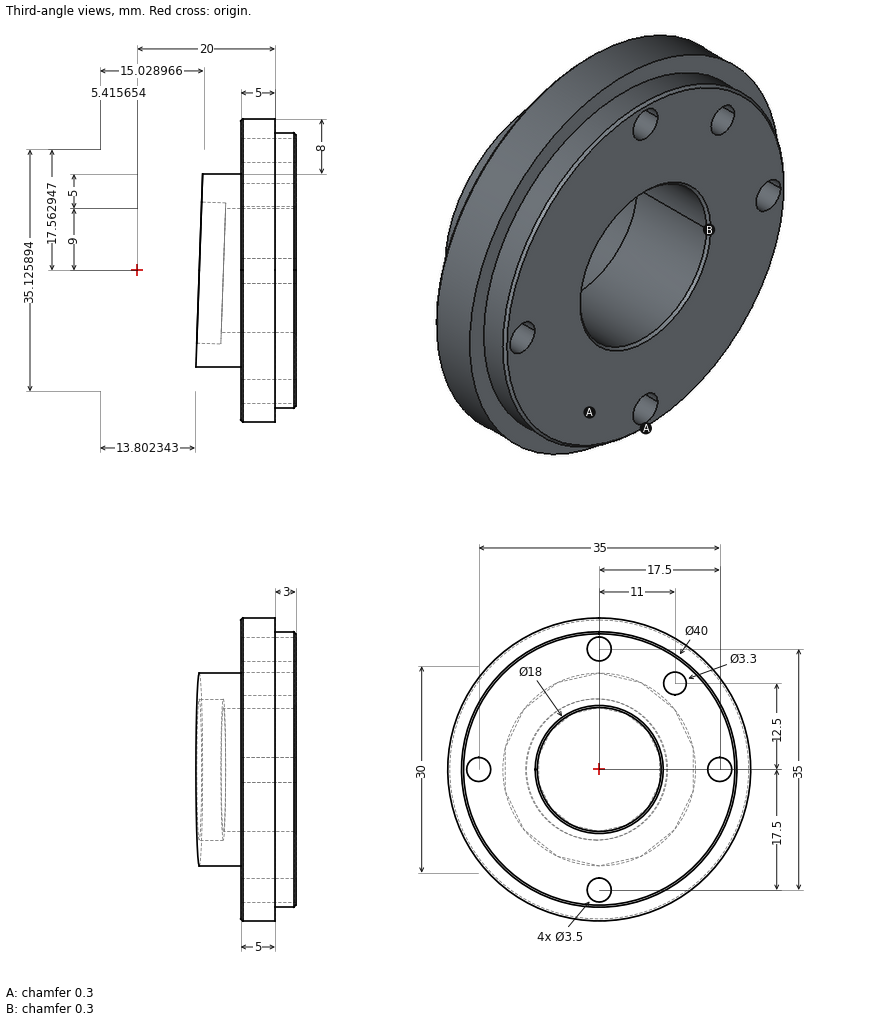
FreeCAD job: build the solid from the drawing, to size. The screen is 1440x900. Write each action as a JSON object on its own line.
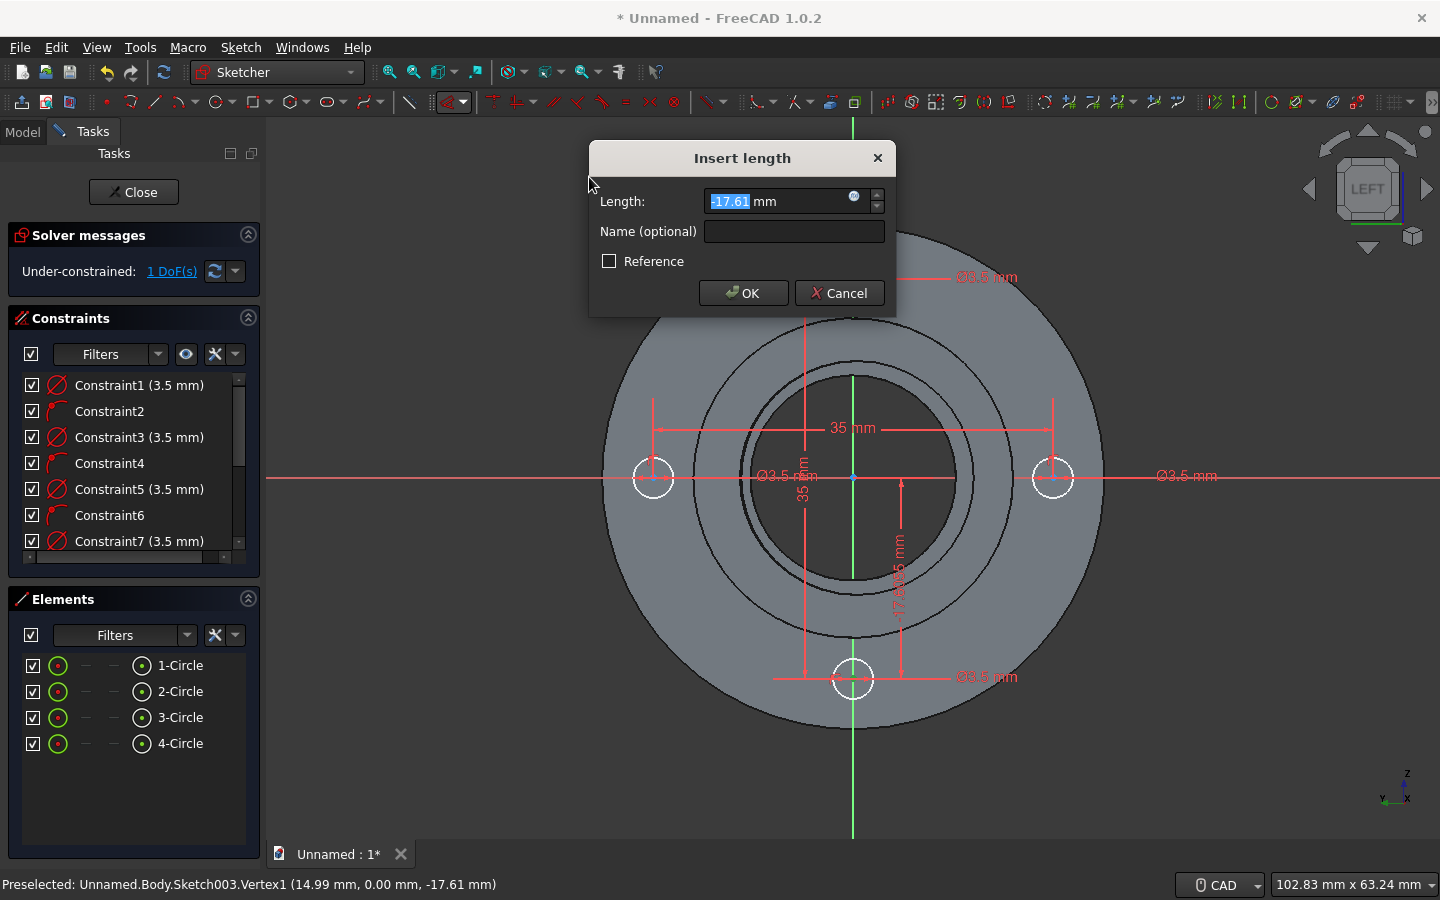
{"action": "type", "text": "-17.5"}
{"action": "key", "text": "Return"}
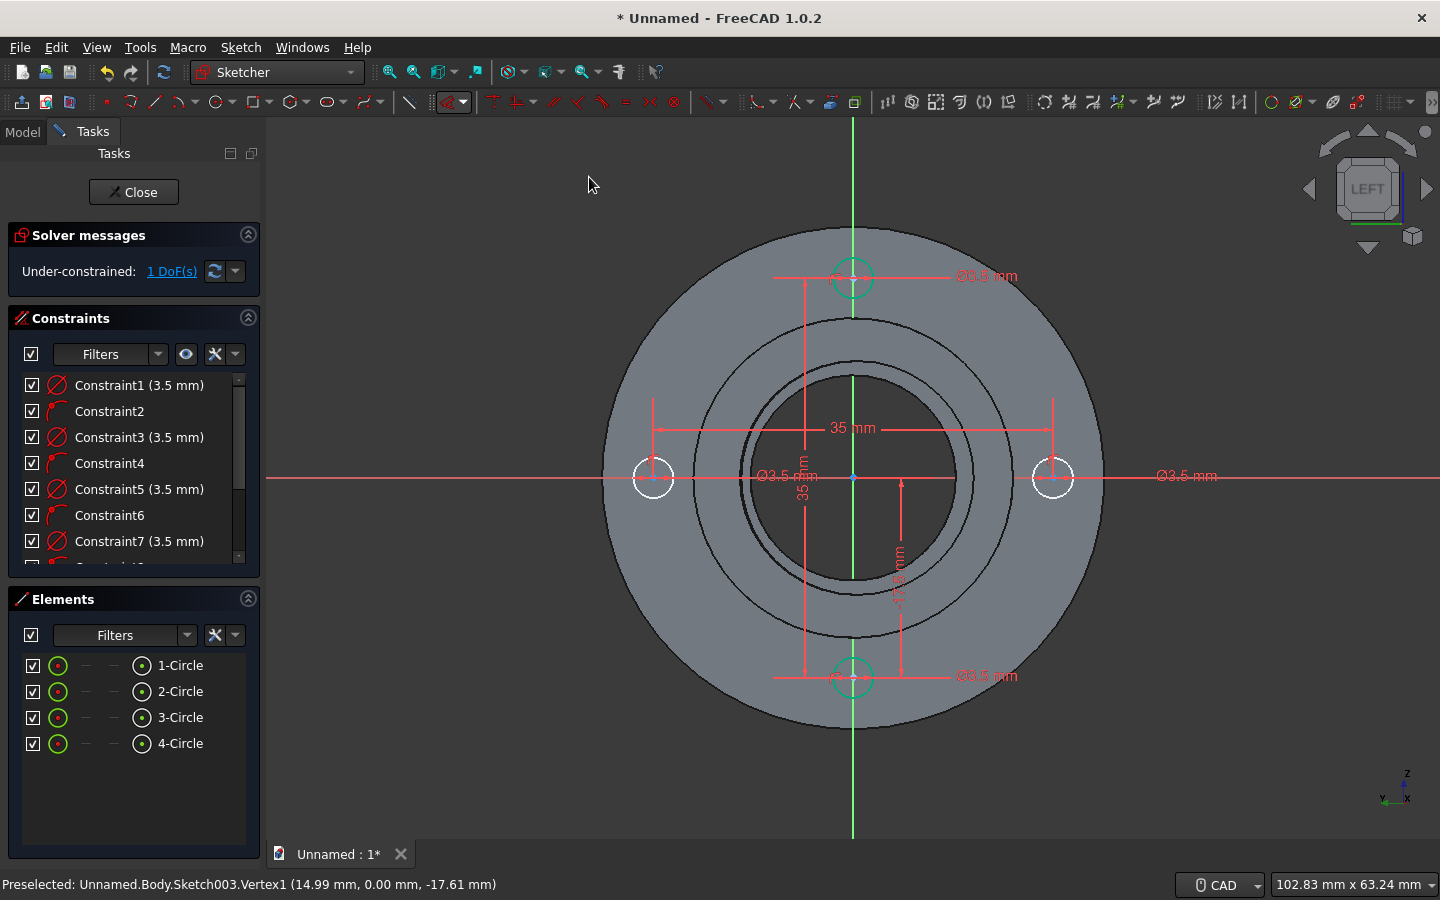
{"action": "left_click", "coordinate": [653, 478]}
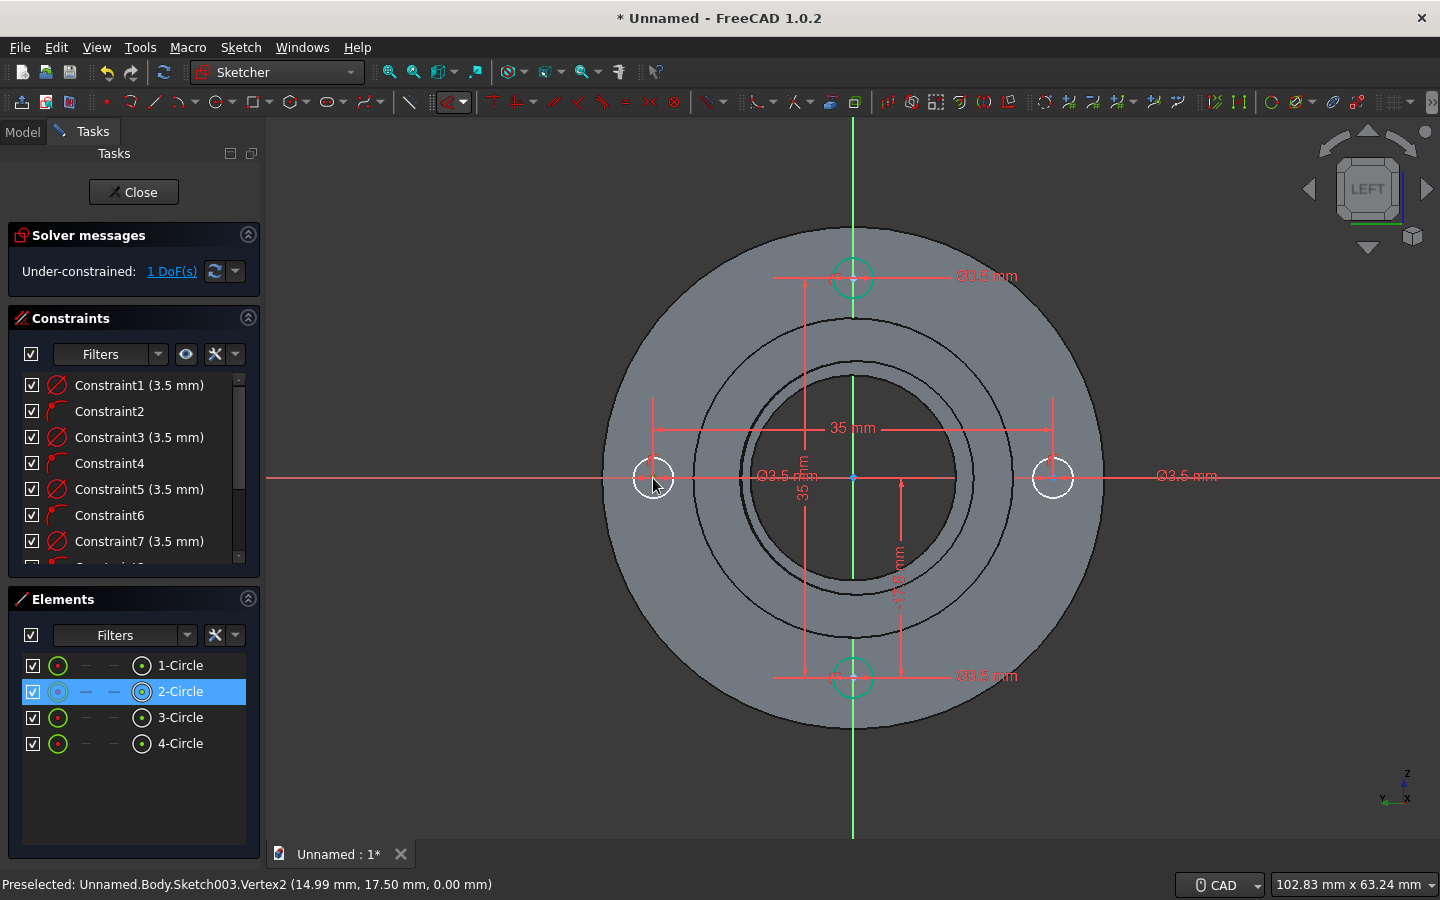
{"action": "key", "text": "l"}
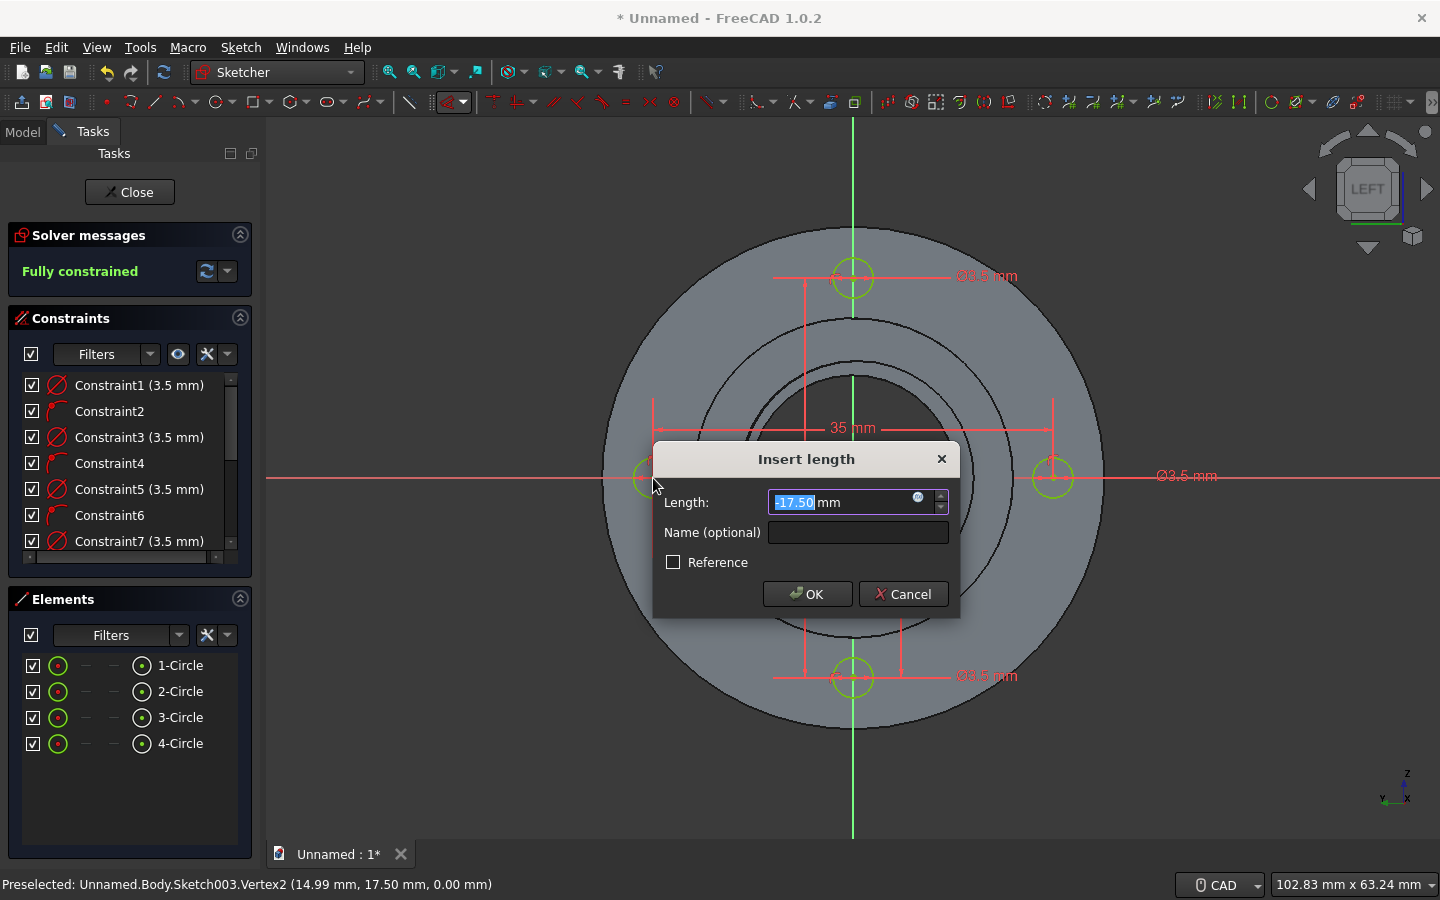
{"action": "type", "text": "-17.5"}
{"action": "key", "text": "Return"}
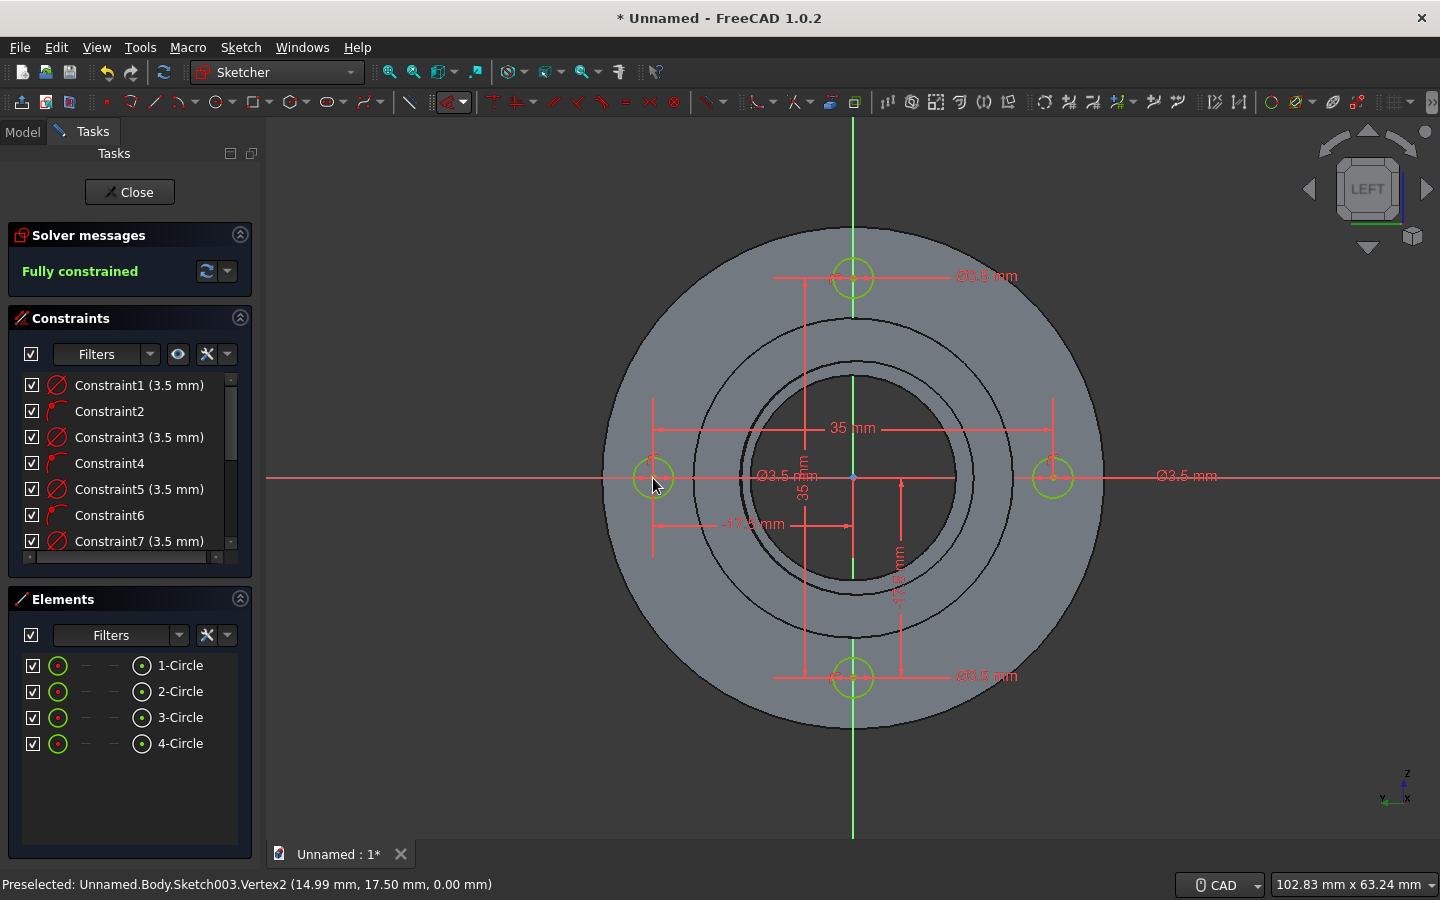
{"action": "left_click", "coordinate": [130, 192]}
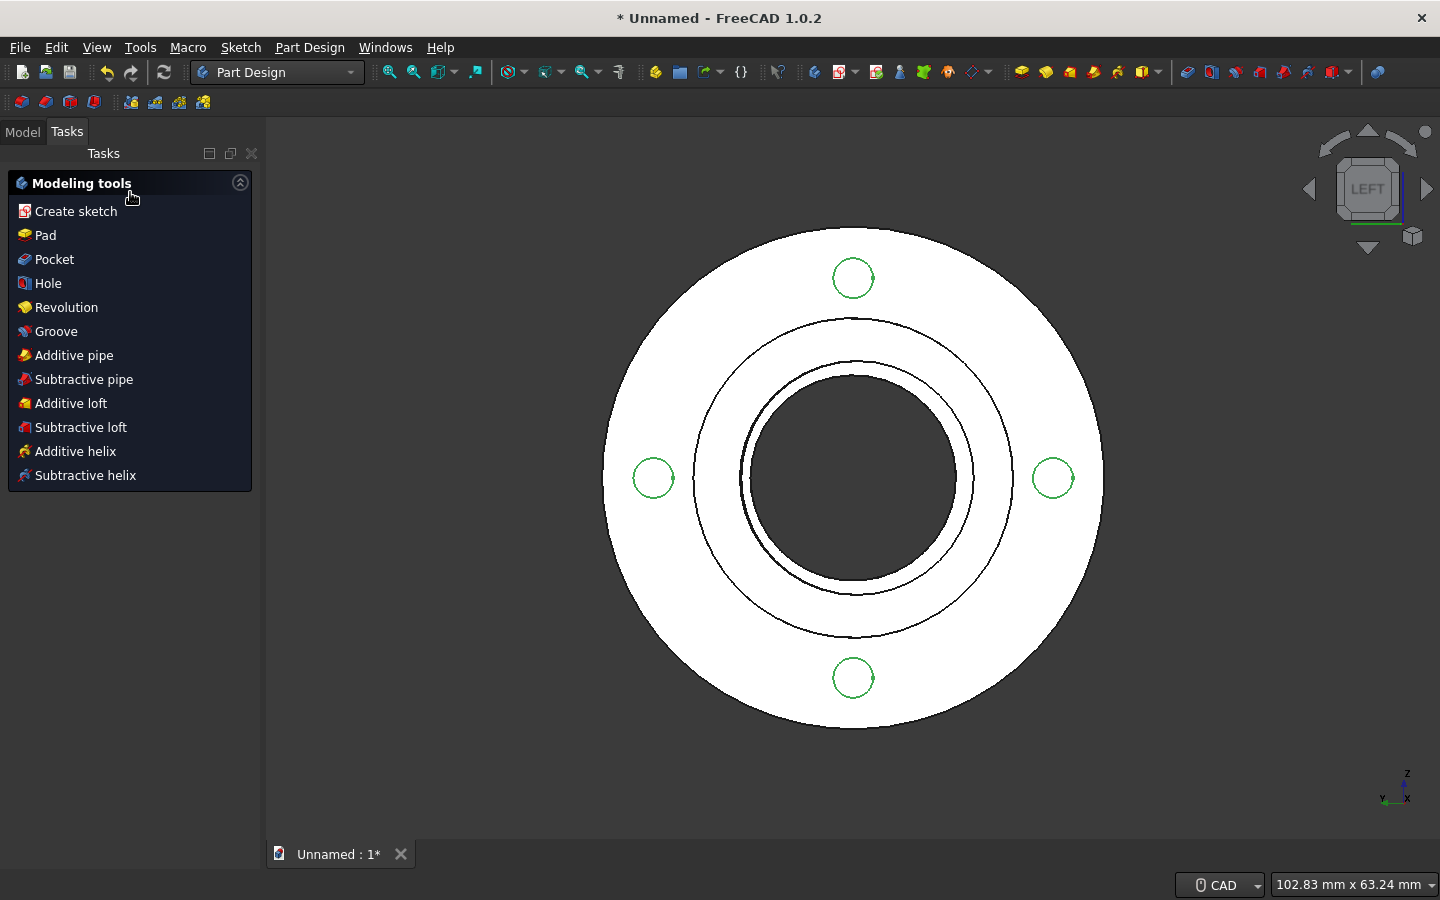
{"action": "left_click", "coordinate": [1188, 72]}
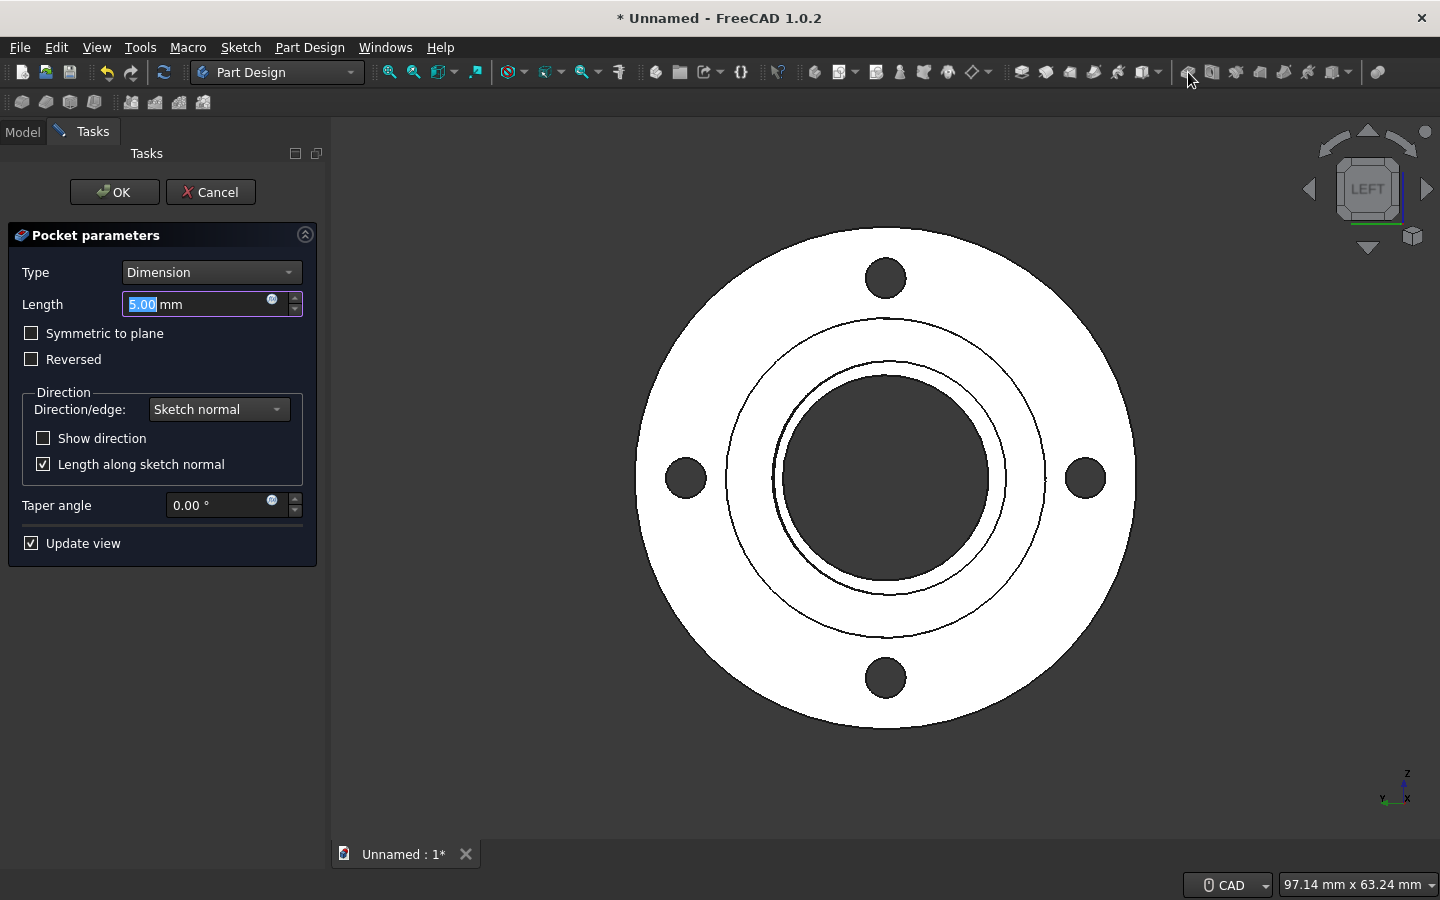
{"action": "type", "text": "5"}
{"action": "key", "text": "Tab"}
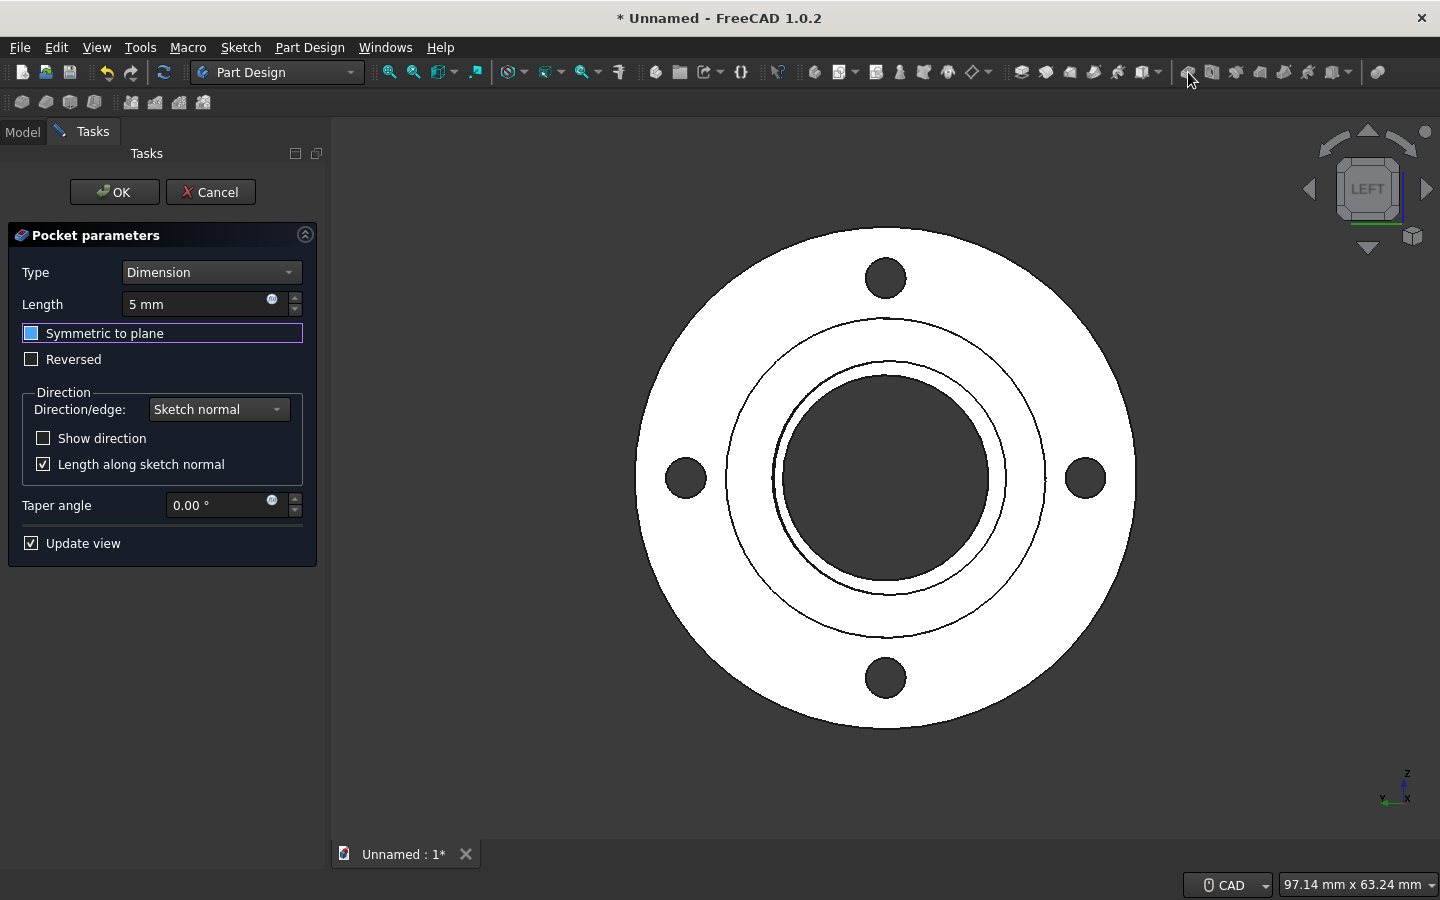
{"action": "left_click", "coordinate": [115, 192]}